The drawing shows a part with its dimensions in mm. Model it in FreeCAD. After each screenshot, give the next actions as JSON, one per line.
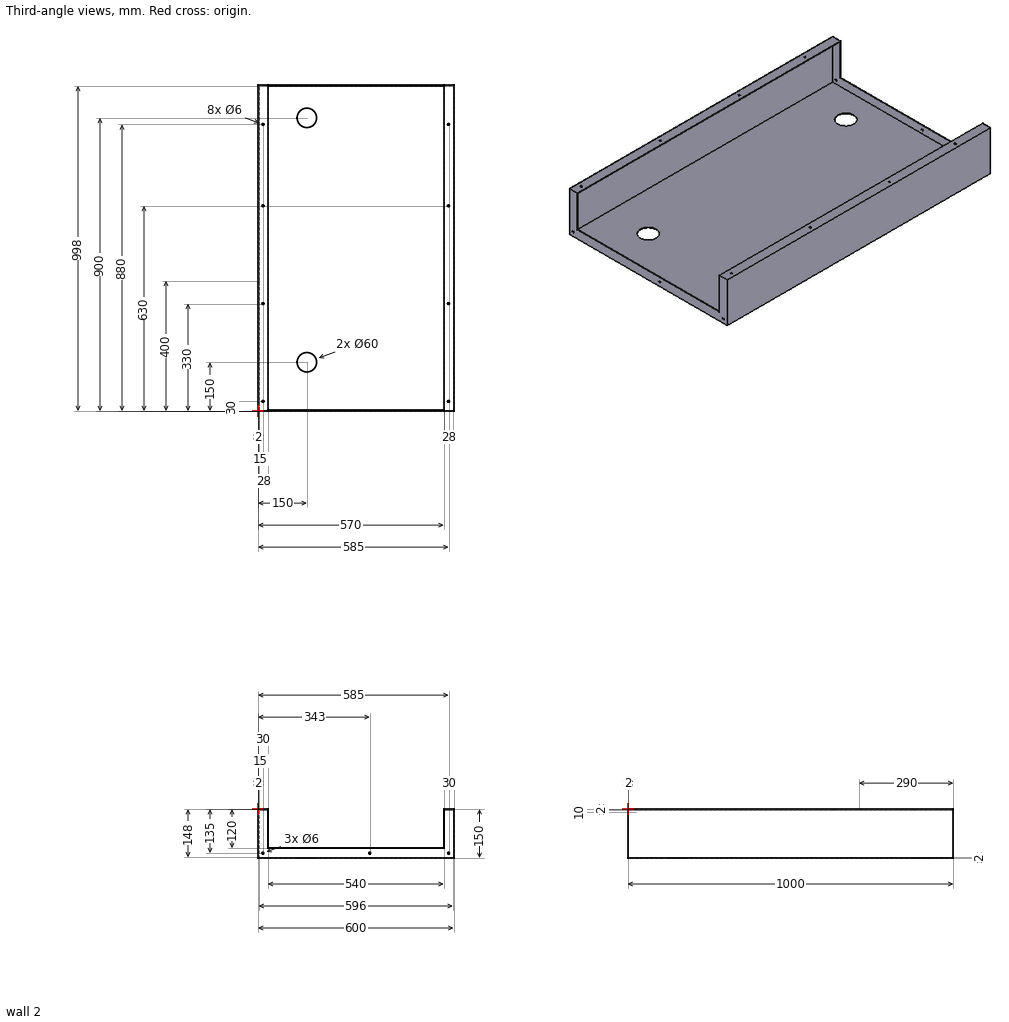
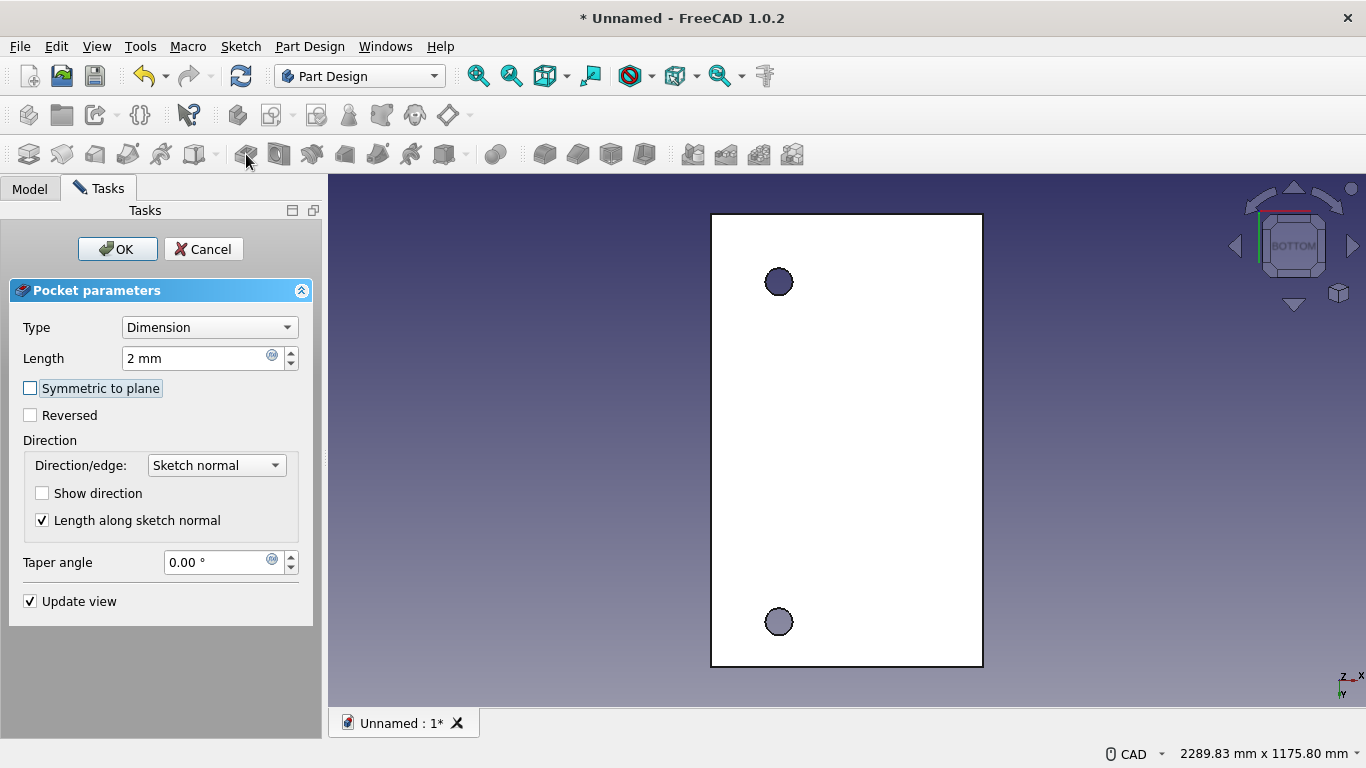
{"action": "left_click", "coordinate": [118, 249]}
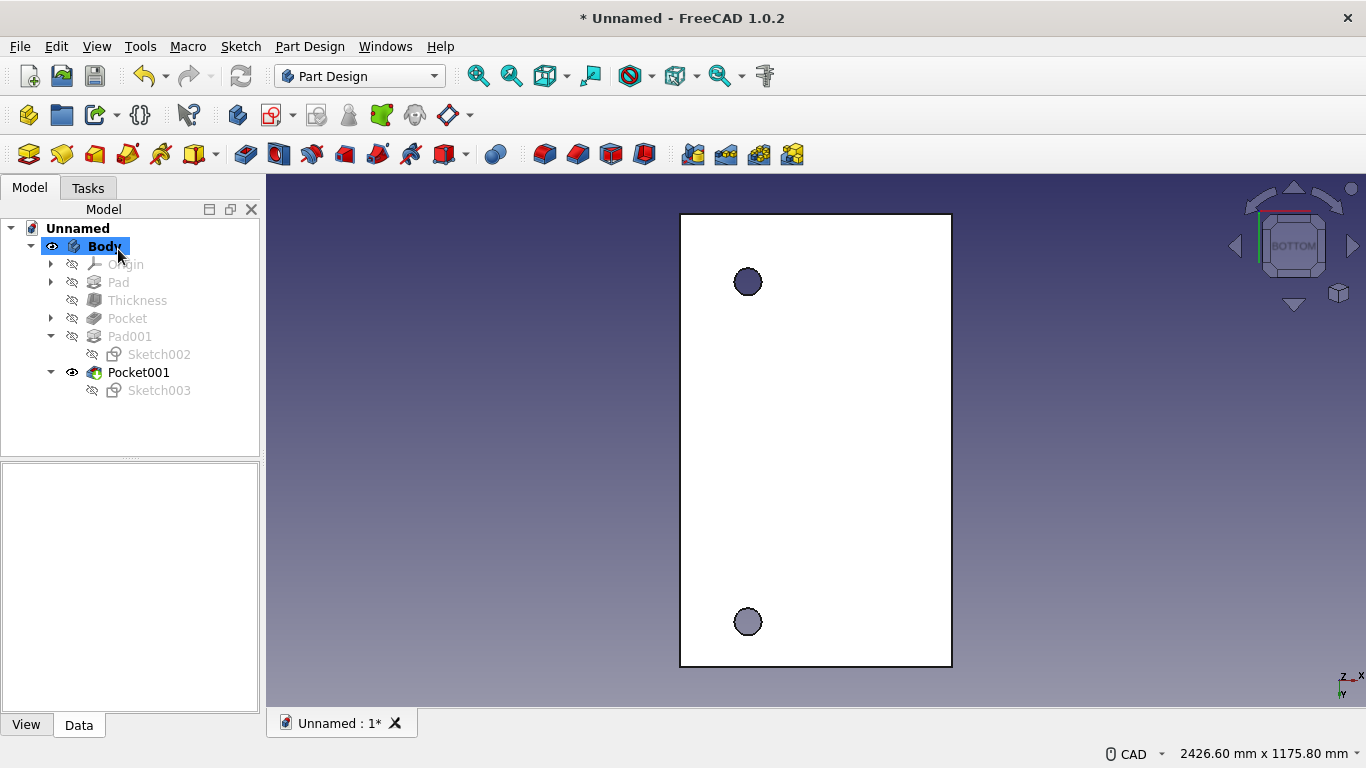
{"action": "key", "text": "4"}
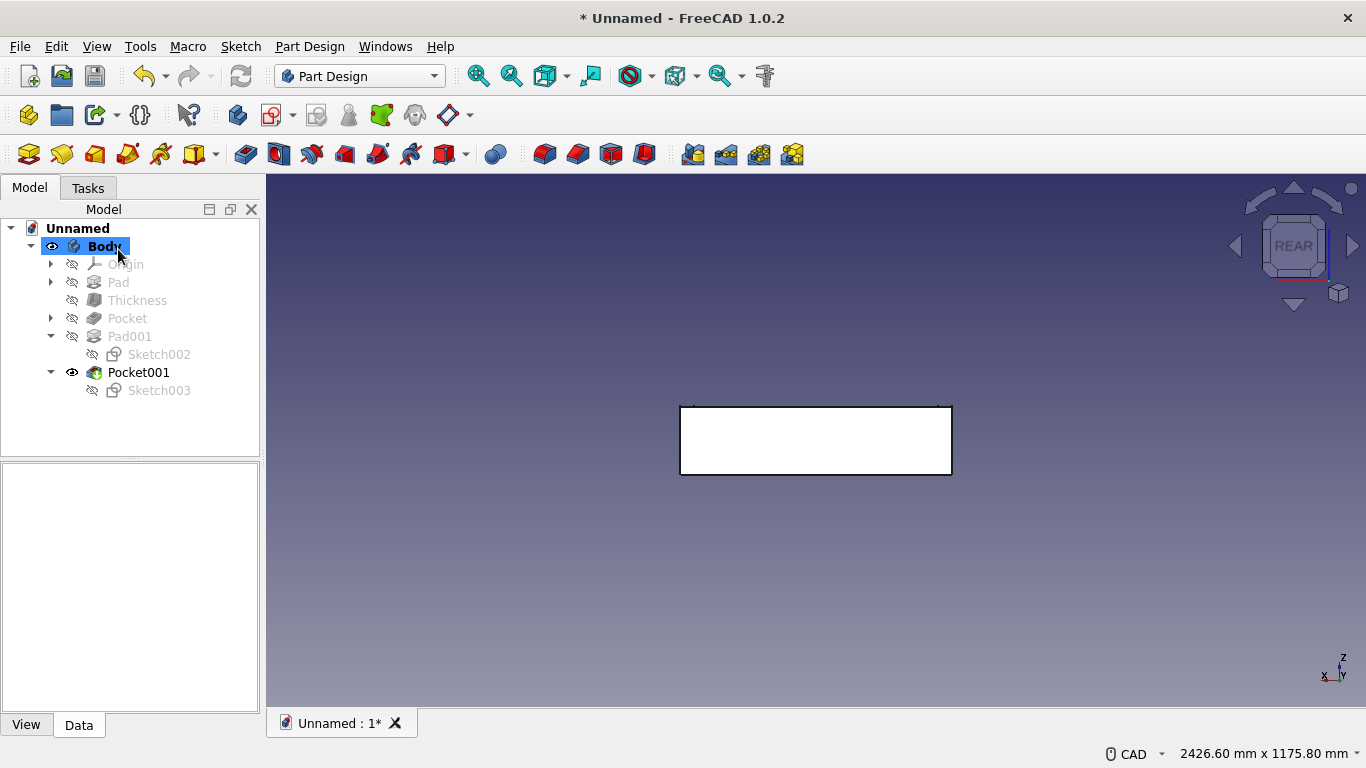
{"action": "left_click", "coordinate": [479, 76]}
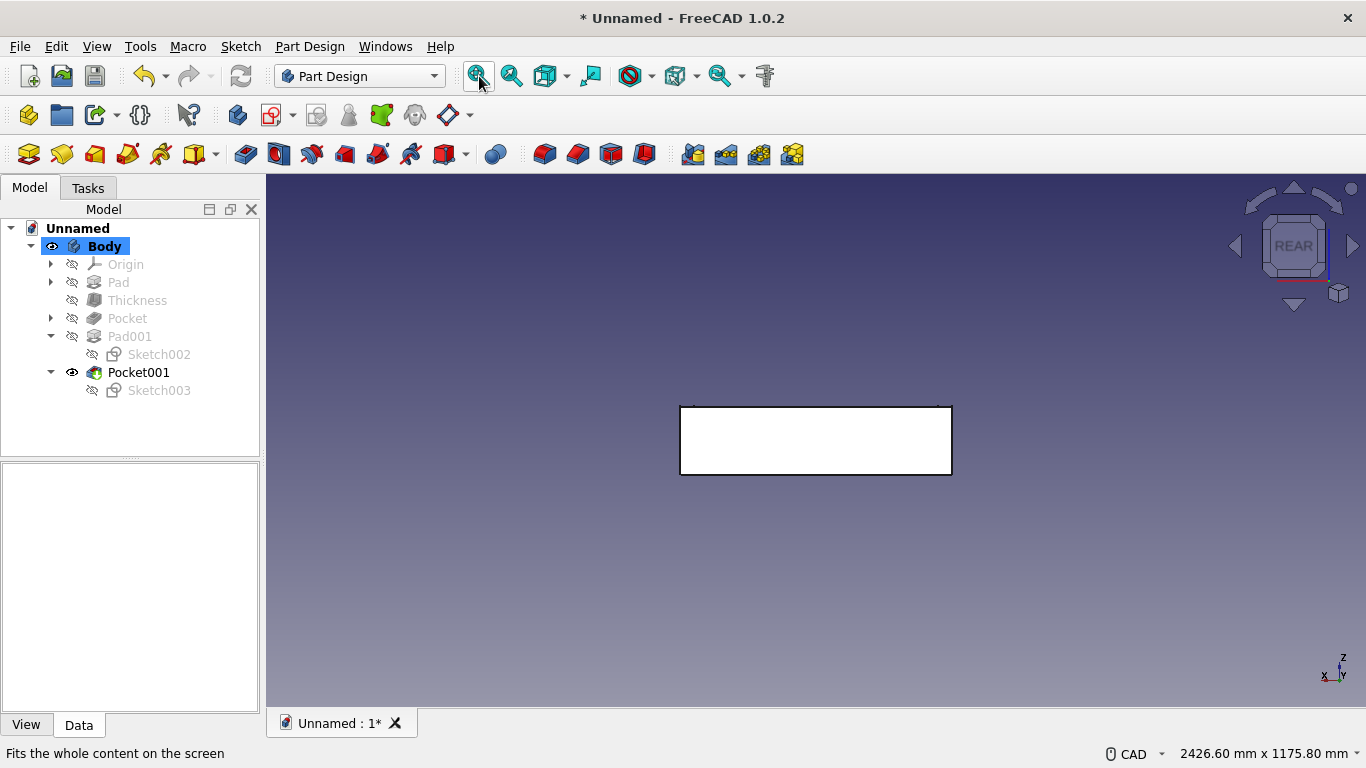
{"action": "left_click", "coordinate": [738, 440]}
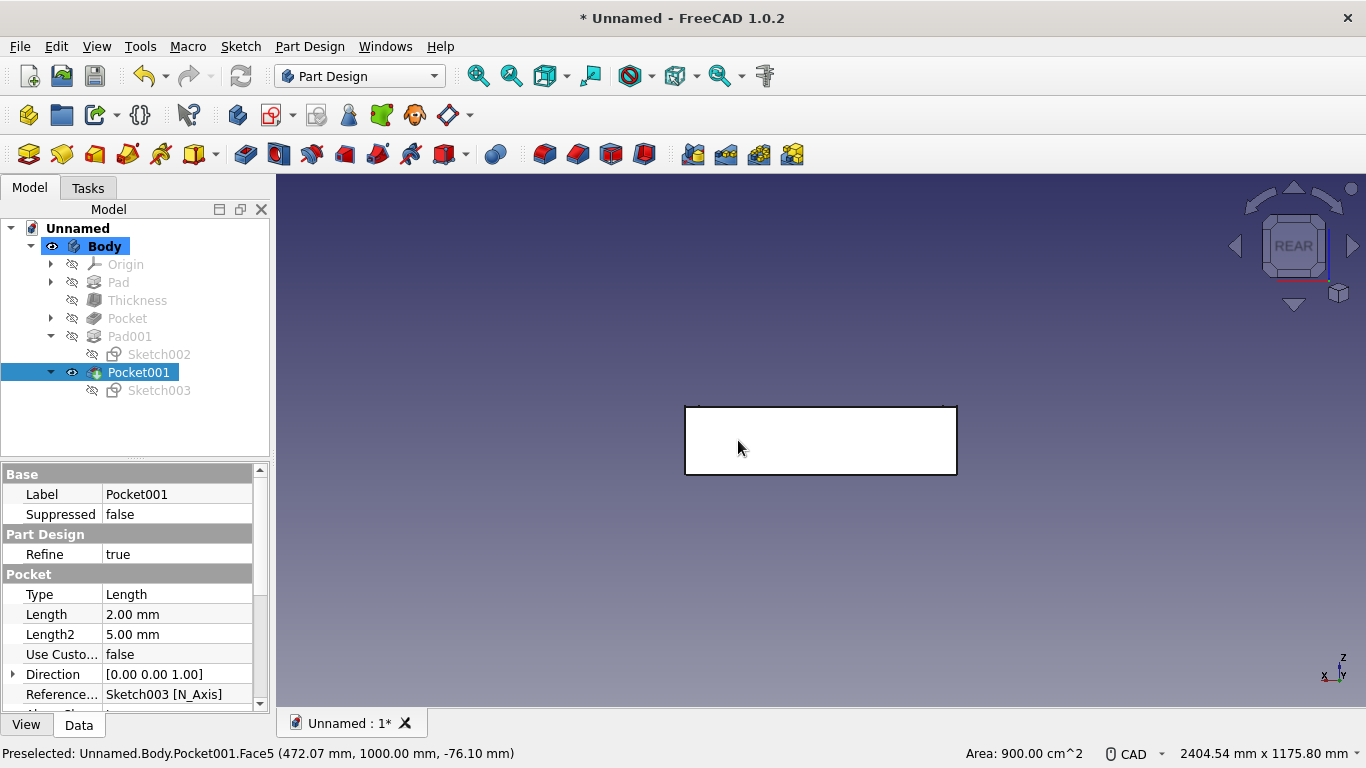
{"action": "left_click", "coordinate": [270, 116]}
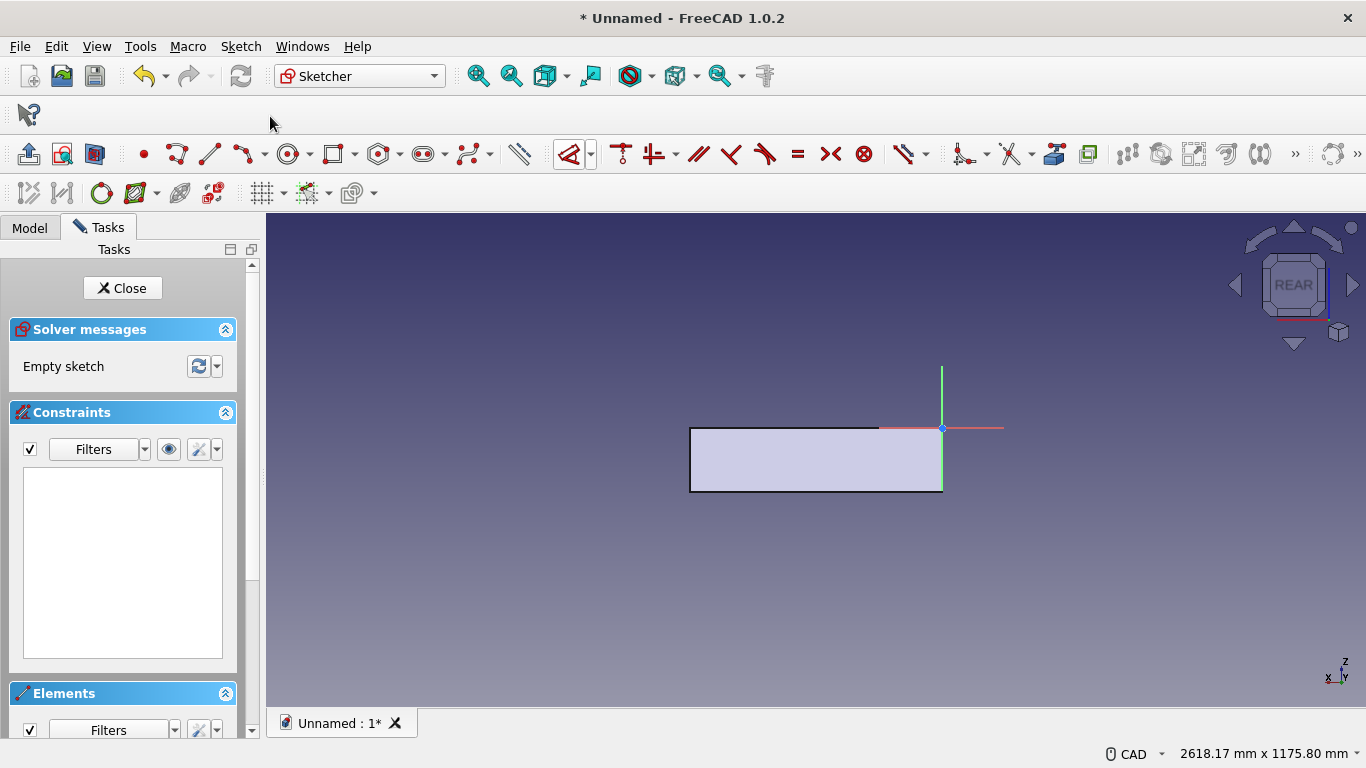
{"action": "scroll", "coordinate": [866, 450], "scroll_direction": "up", "scroll_amount": 5}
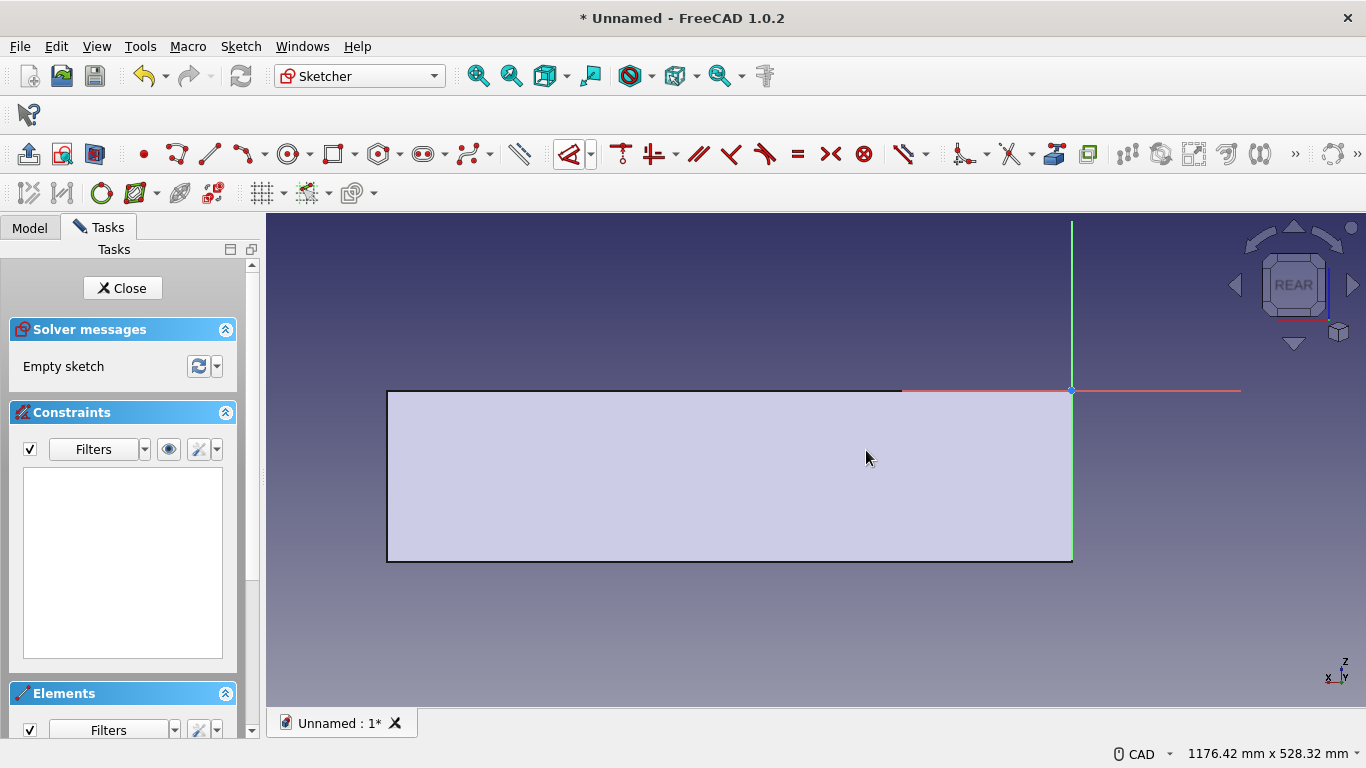
{"action": "left_click", "coordinate": [332, 154]}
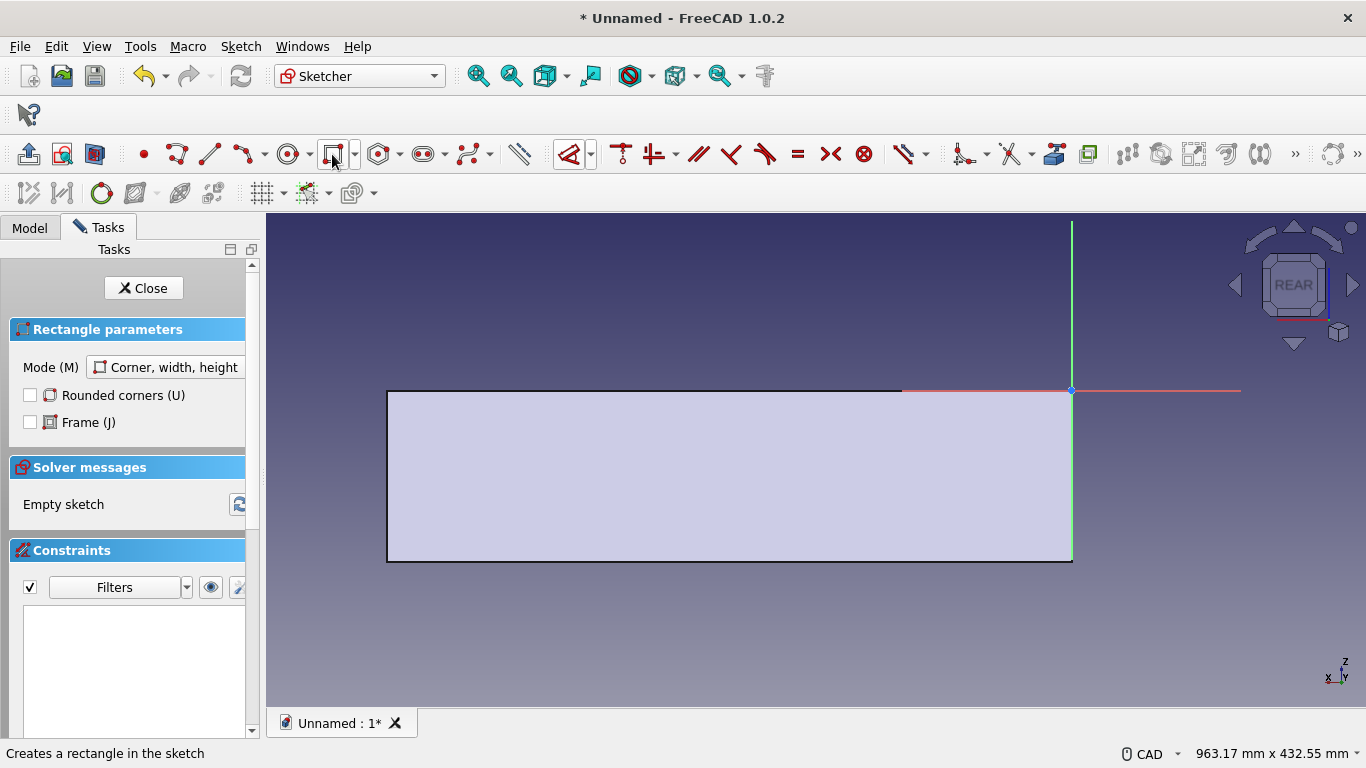
{"action": "left_click", "coordinate": [421, 391]}
{"action": "mouse_move", "coordinate": [1038, 528]}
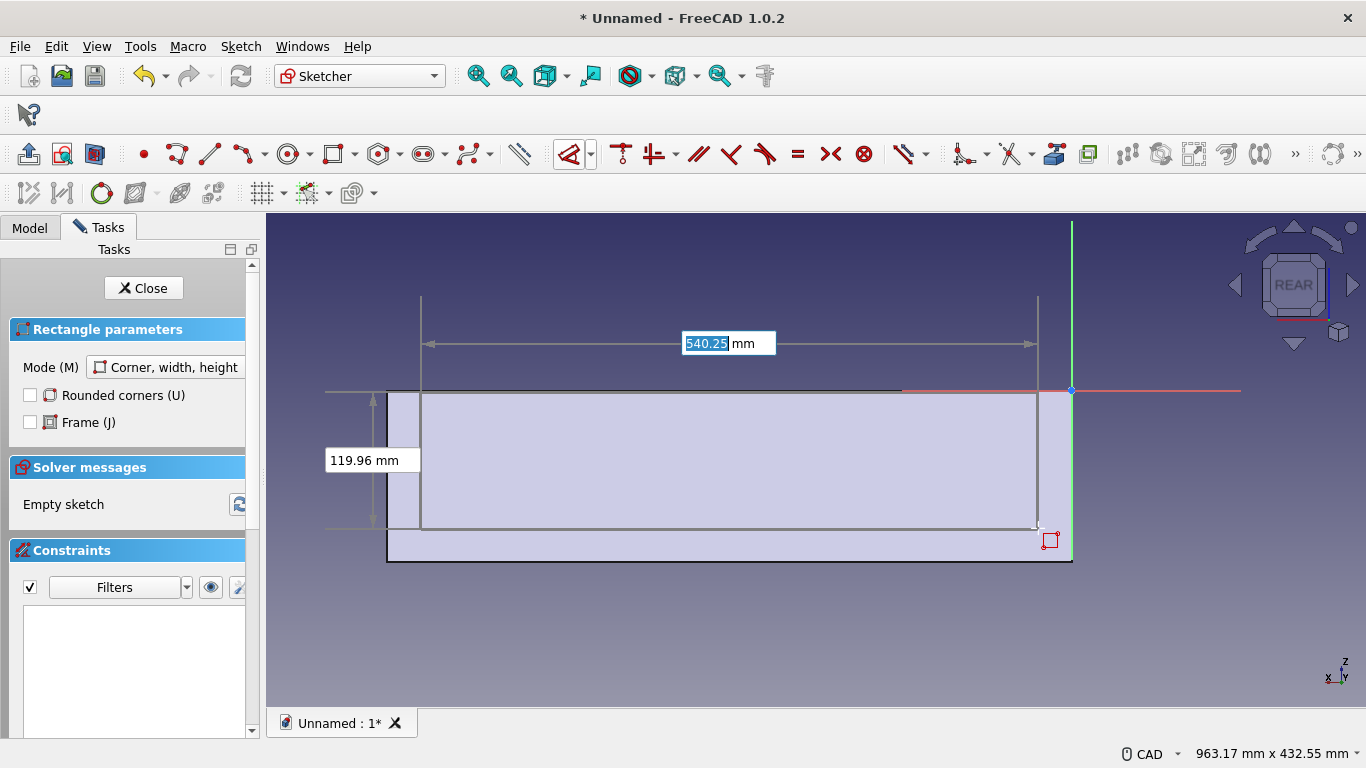
{"action": "type", "text": "540"}
{"action": "key", "text": "Tab"}
{"action": "type", "text": "120"}
{"action": "key", "text": "Return"}
{"action": "key", "text": "Escape"}